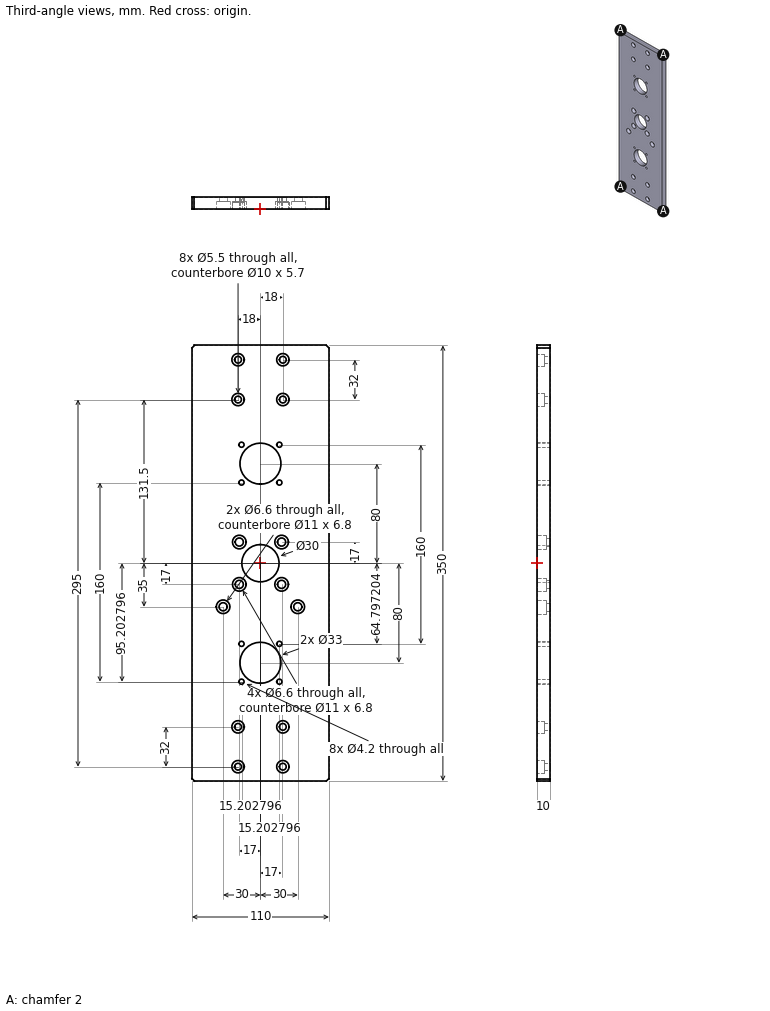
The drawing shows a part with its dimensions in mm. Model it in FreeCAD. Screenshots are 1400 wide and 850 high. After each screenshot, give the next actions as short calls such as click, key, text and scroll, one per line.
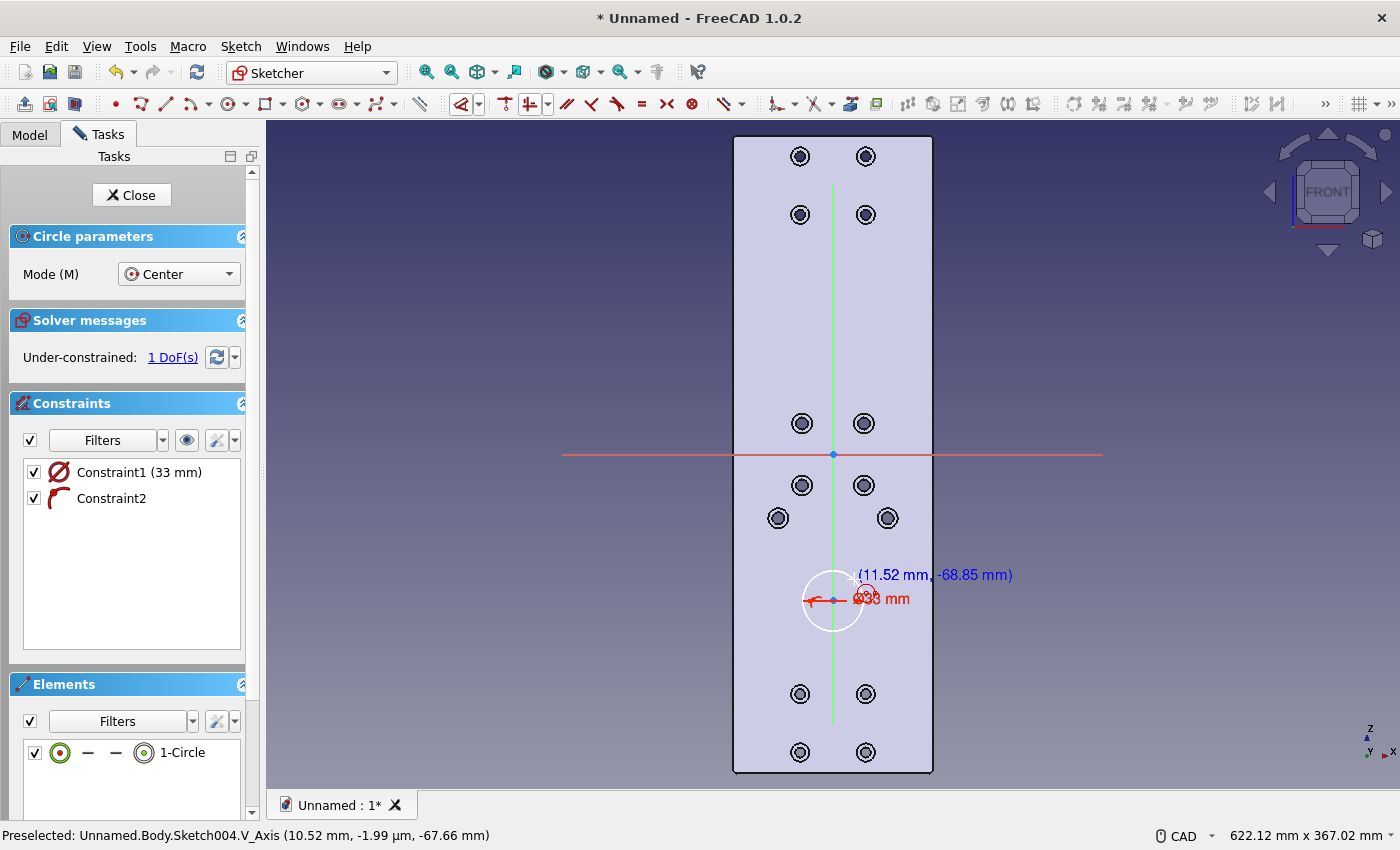
click(833, 309)
move(854, 287)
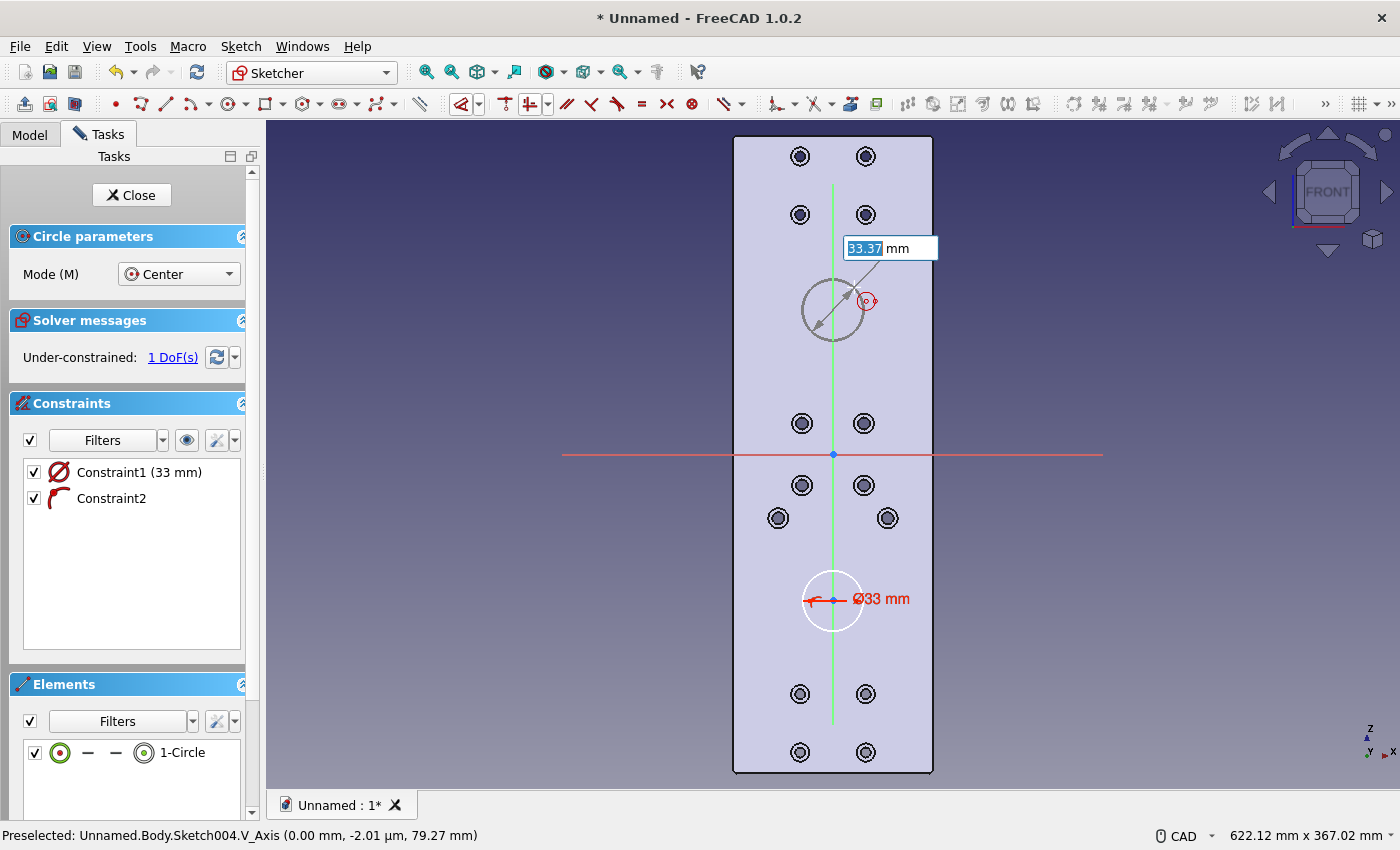
text(33)
key(Return)
key(Escape)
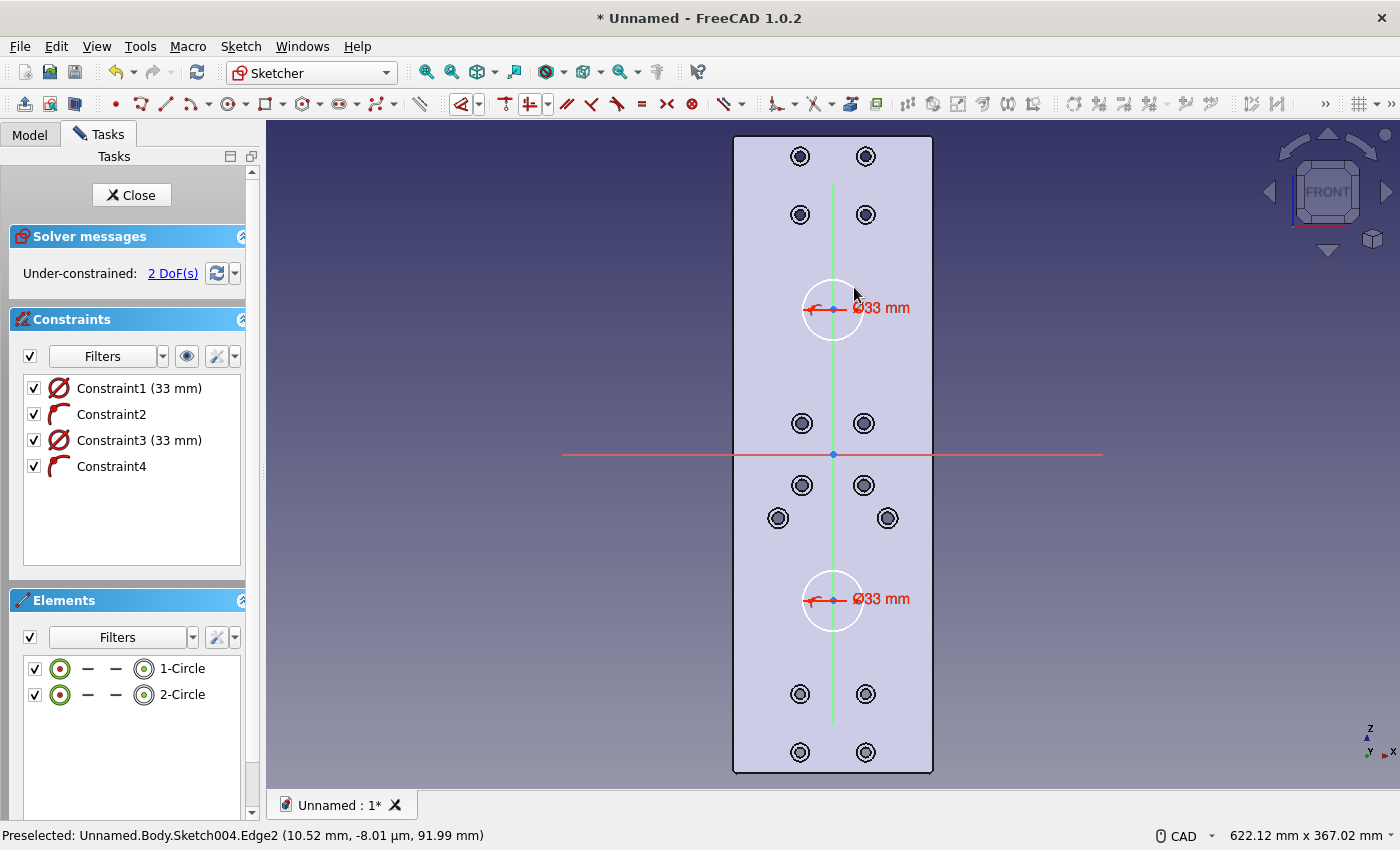
click(833, 601)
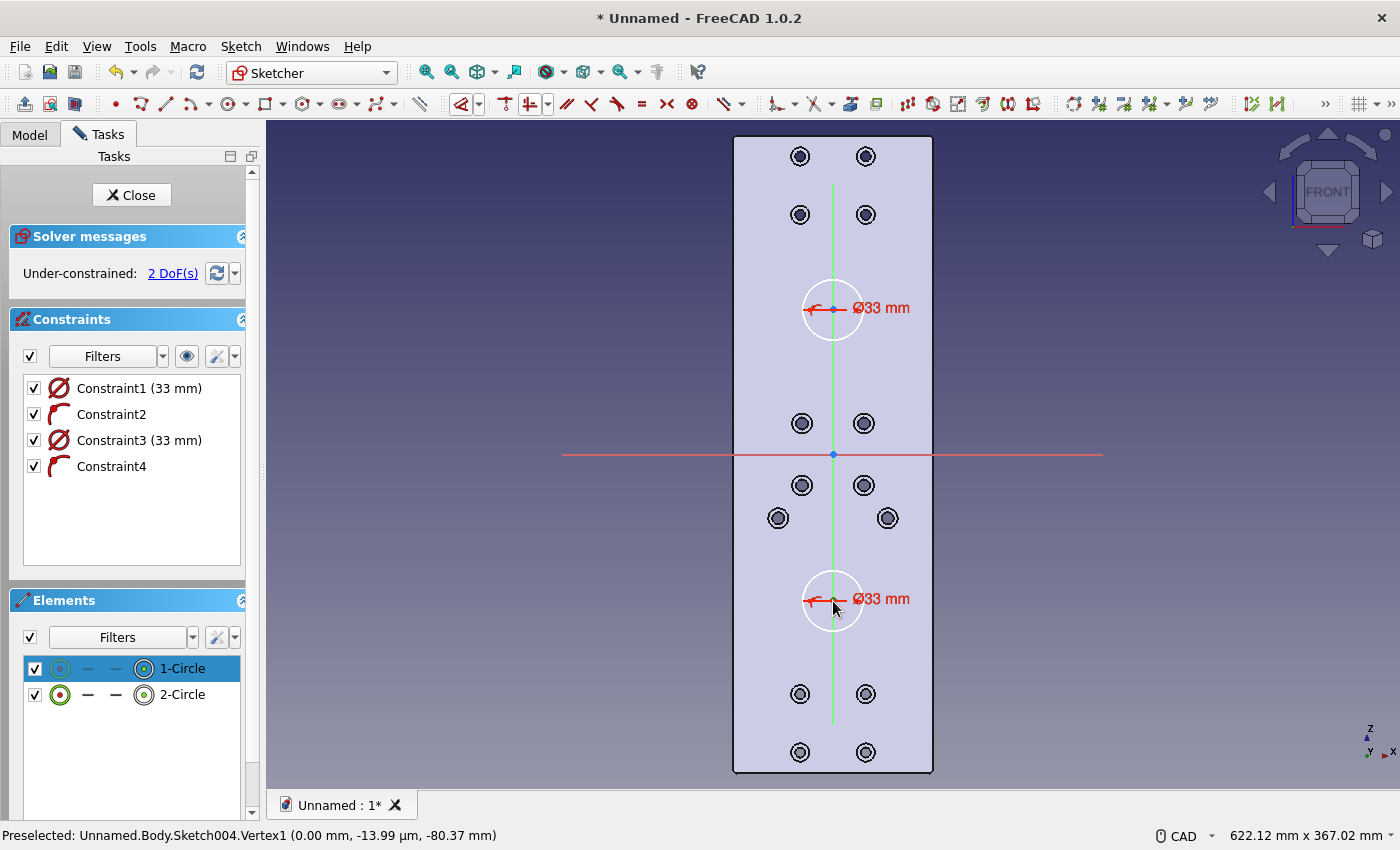
click(478, 104)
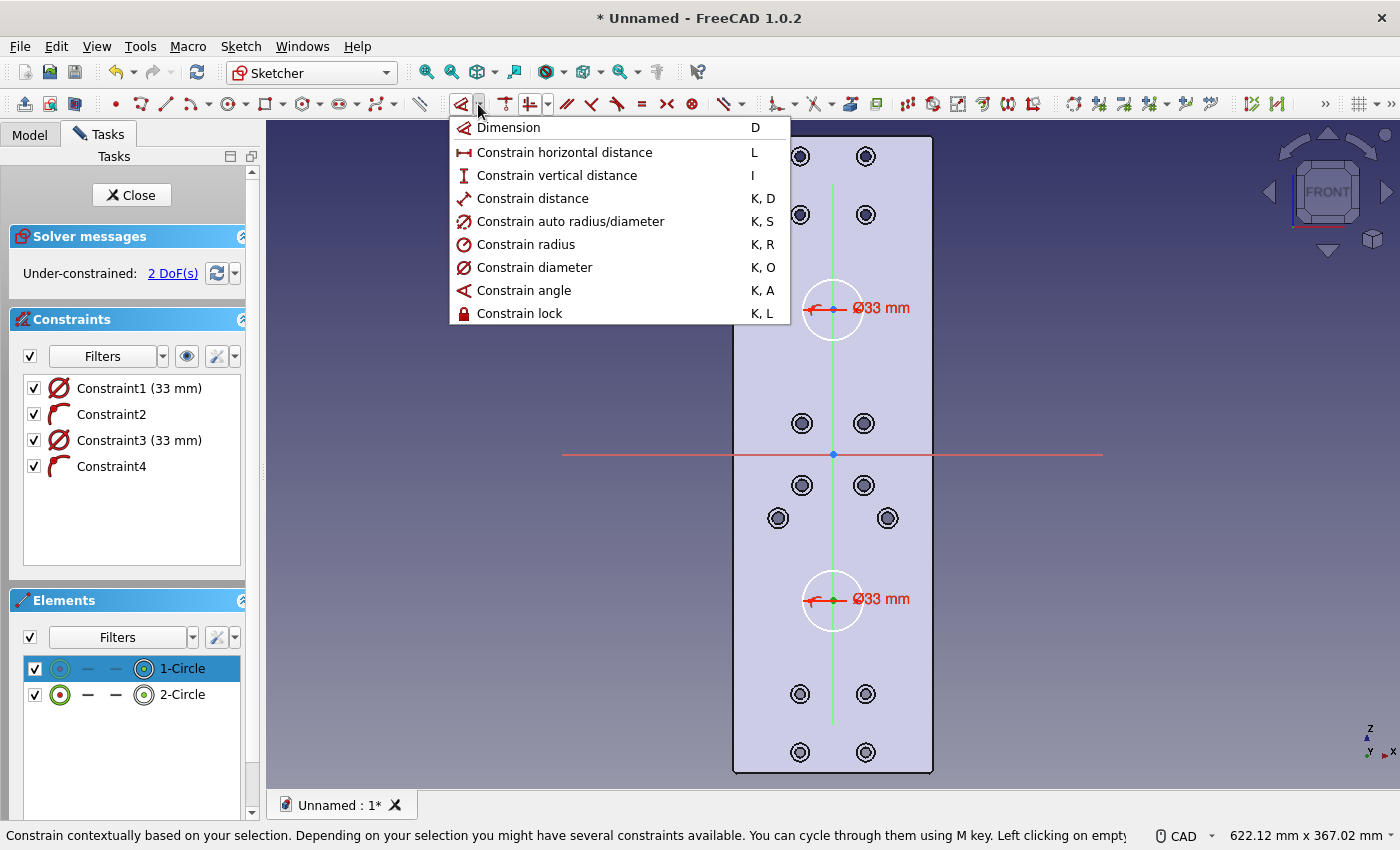
click(620, 176)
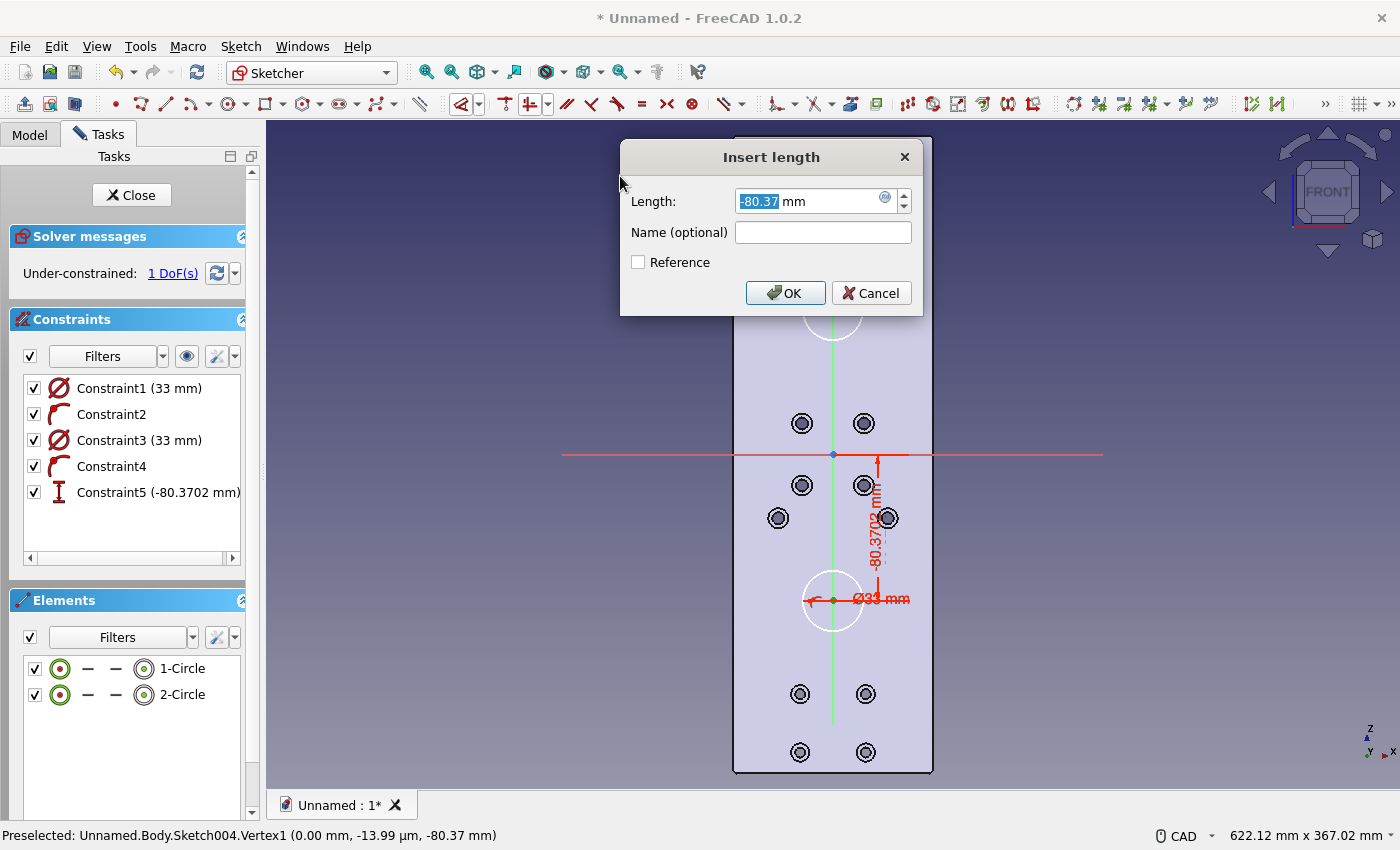
text(-80)
key(Return)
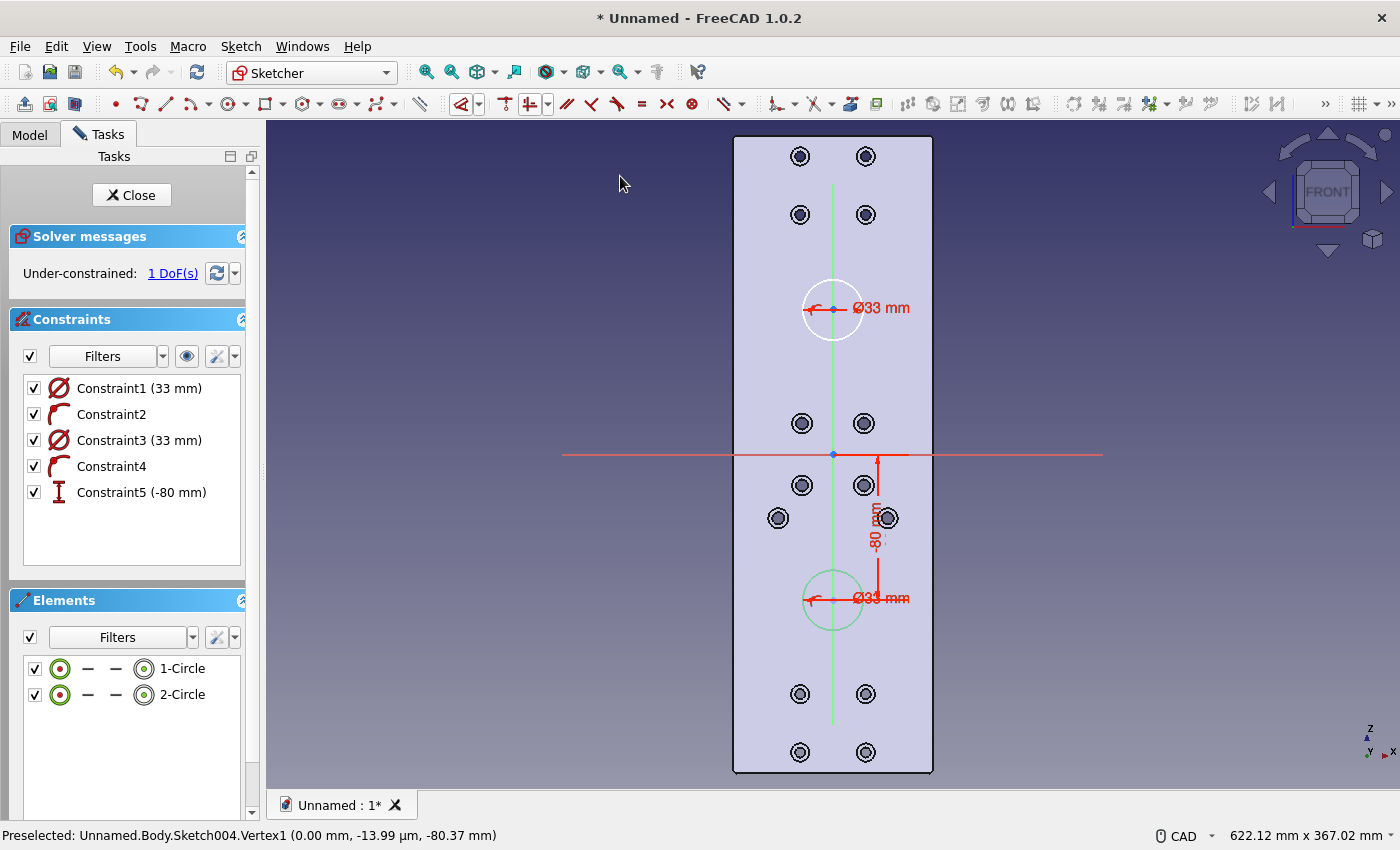
click(833, 310)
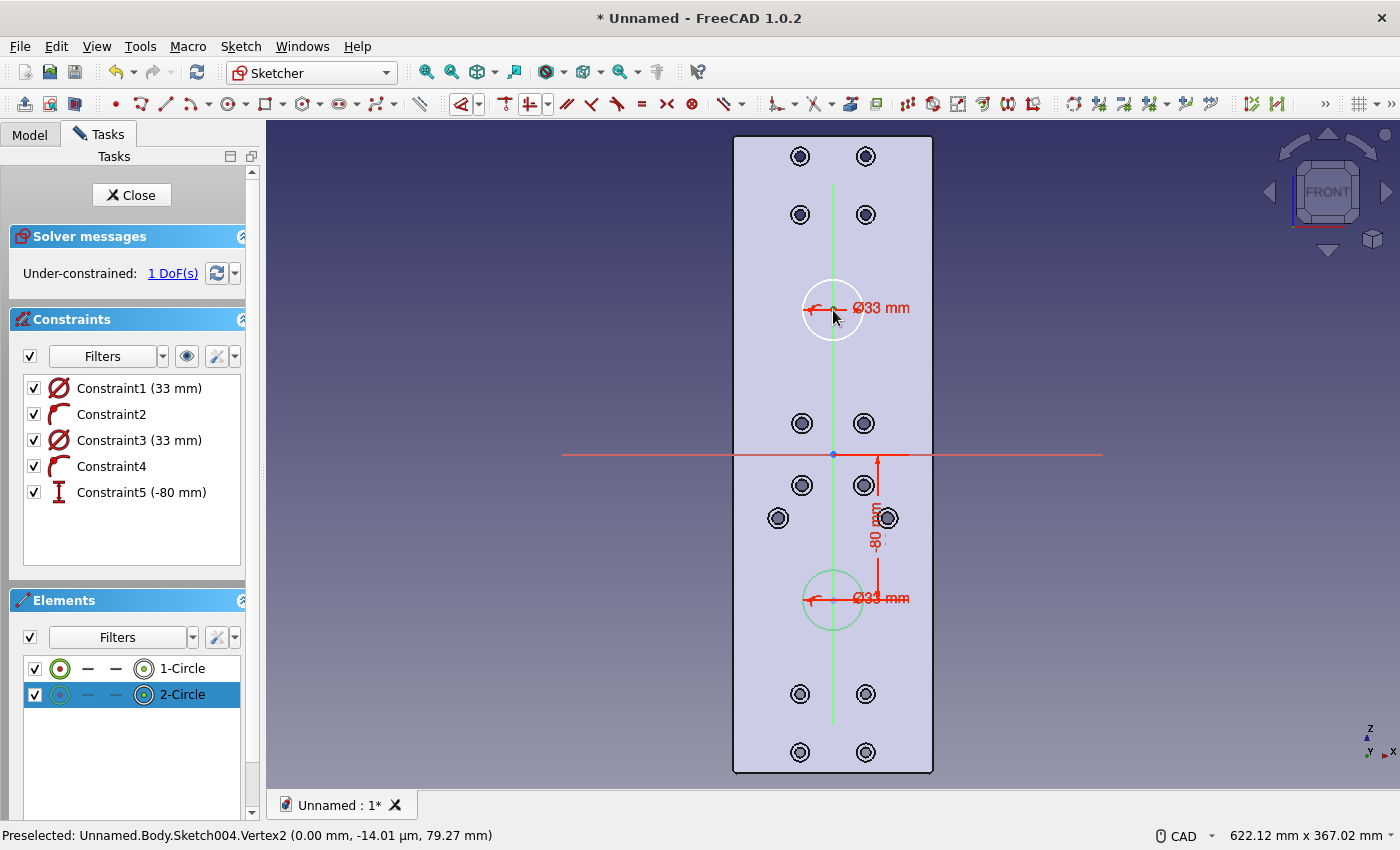
key(i)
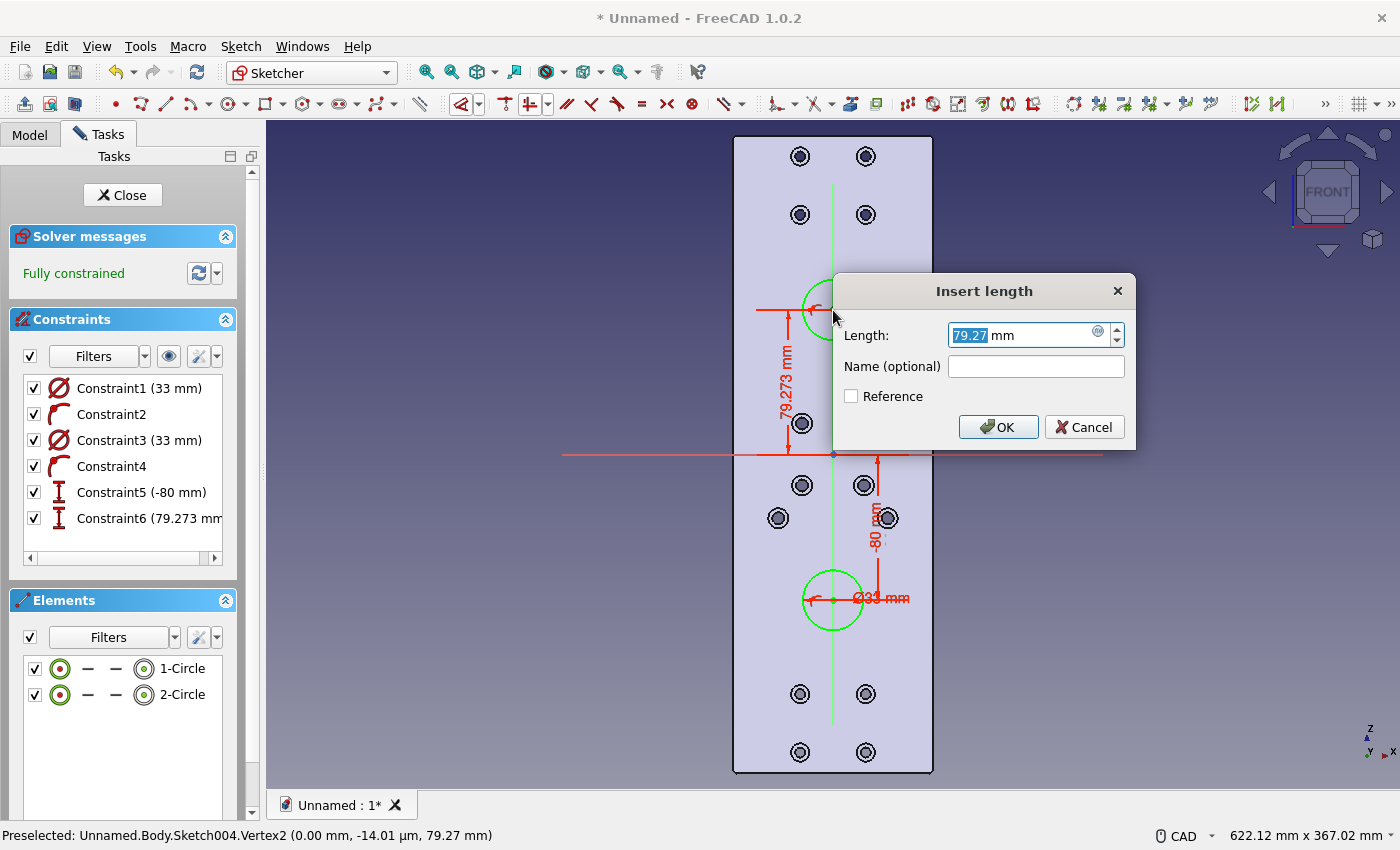
text(80)
key(Return)